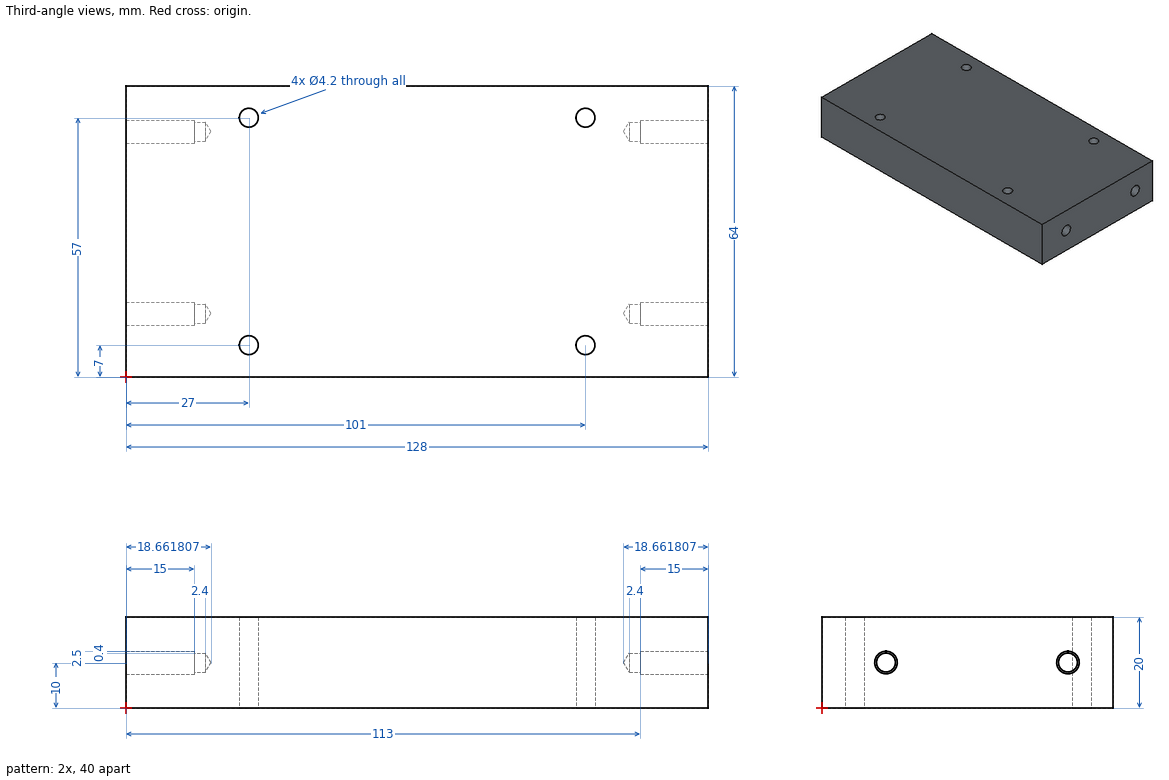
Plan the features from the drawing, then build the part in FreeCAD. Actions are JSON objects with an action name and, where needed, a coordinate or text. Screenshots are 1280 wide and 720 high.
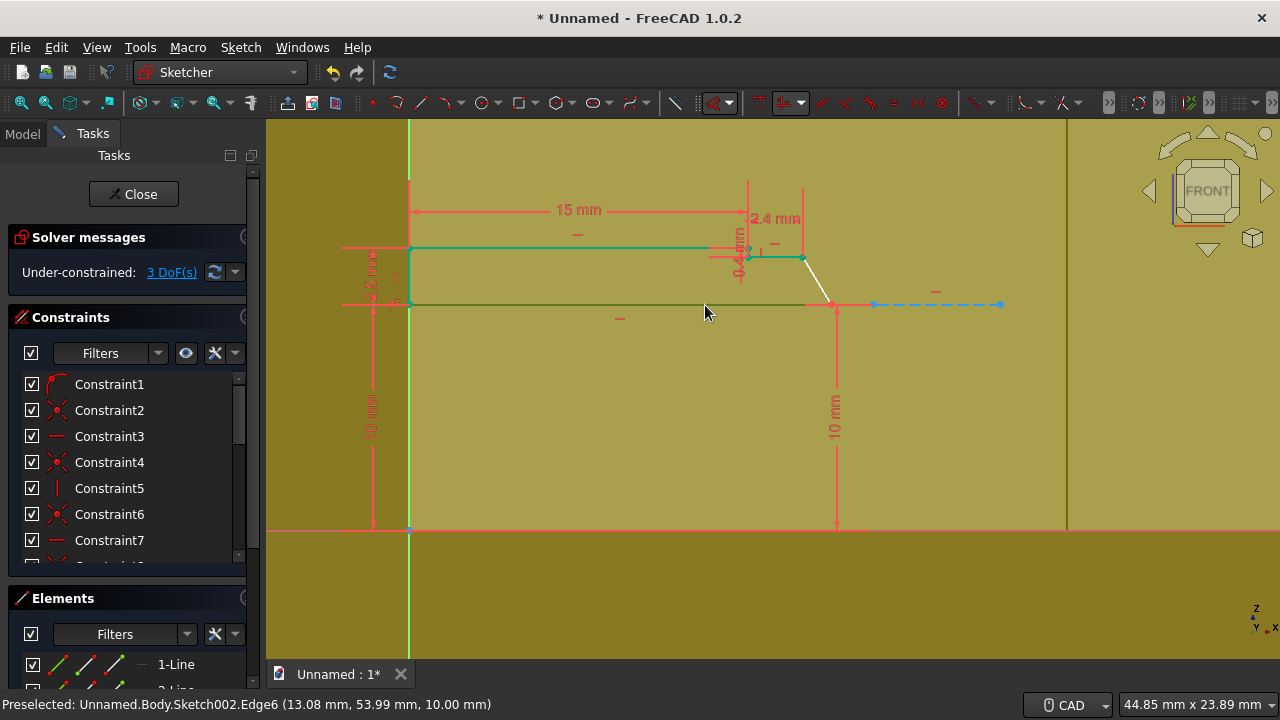
{"action": "left_click", "coordinate": [732, 104]}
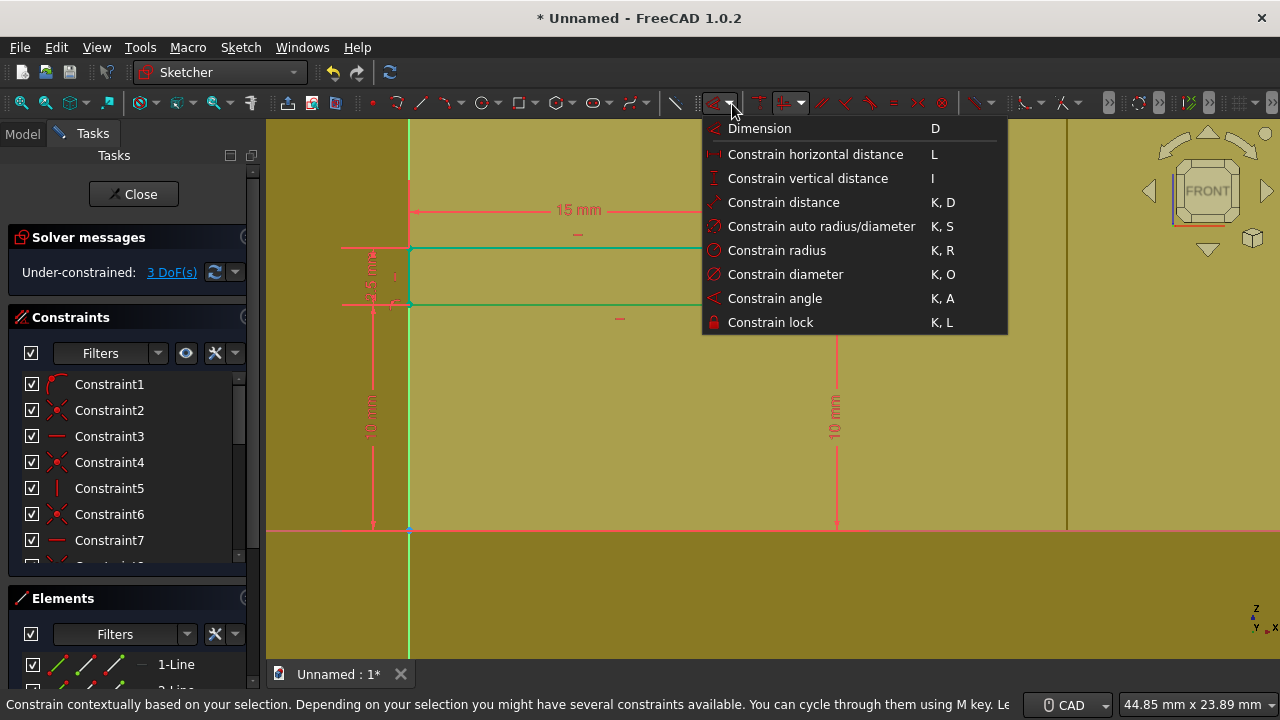
{"action": "left_click", "coordinate": [855, 154]}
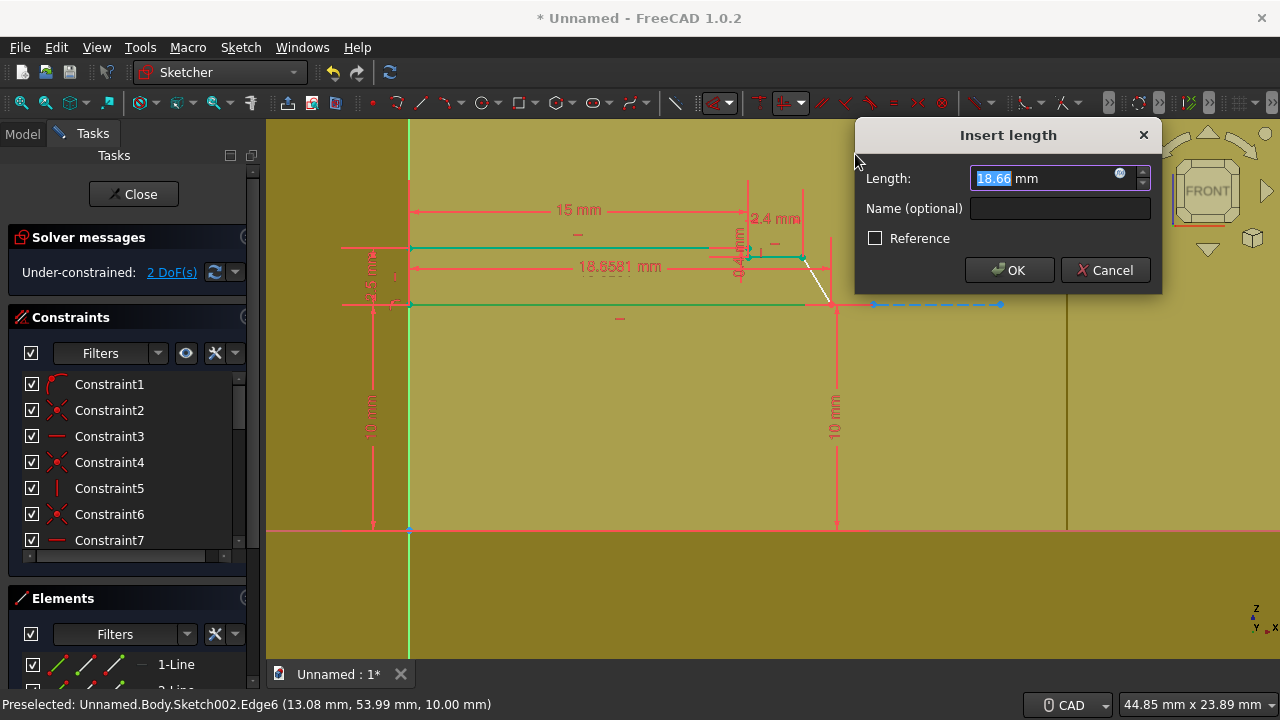
{"action": "type", "text": "18.661807"}
{"action": "key", "text": "Return"}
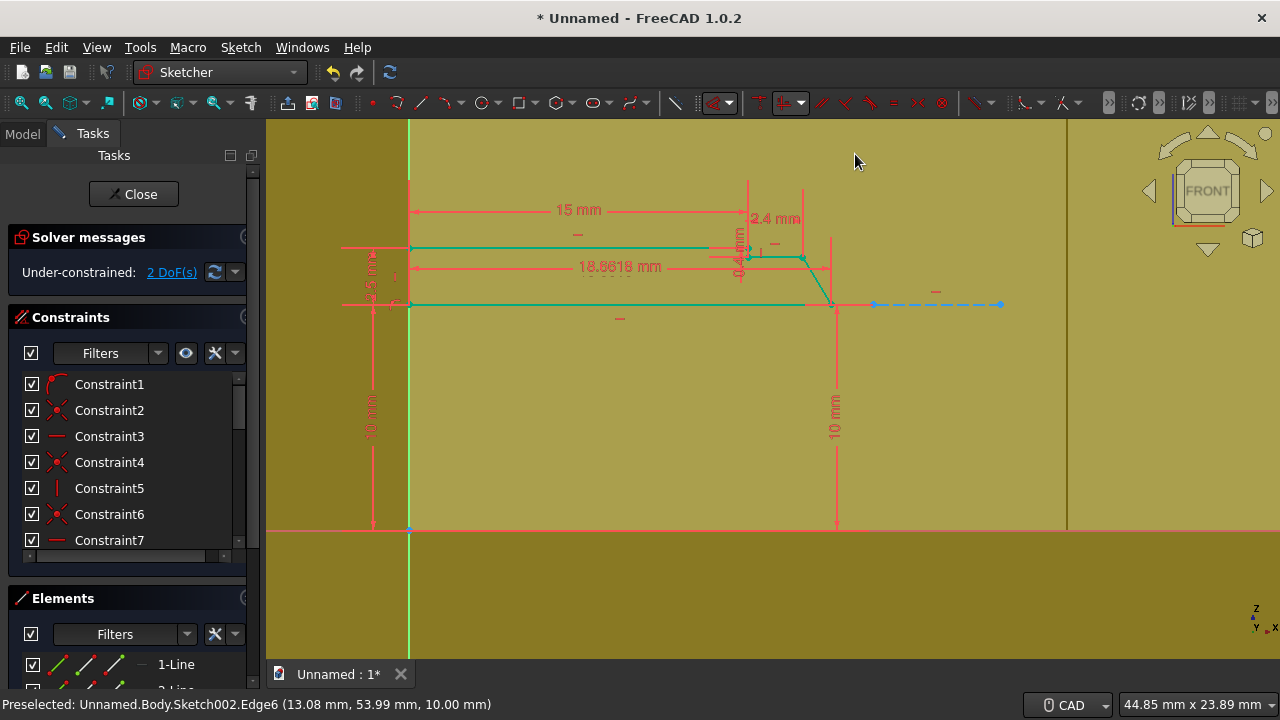
{"action": "left_click", "coordinate": [134, 194]}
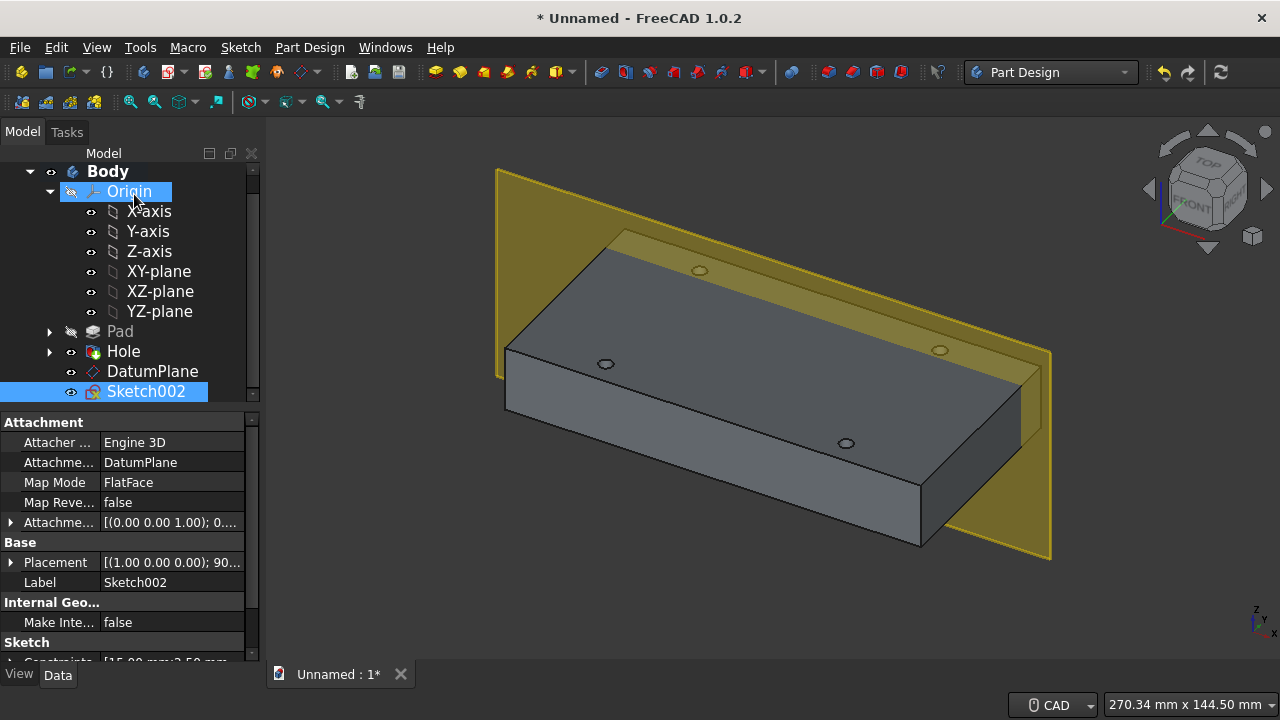
{"action": "left_click", "coordinate": [650, 72]}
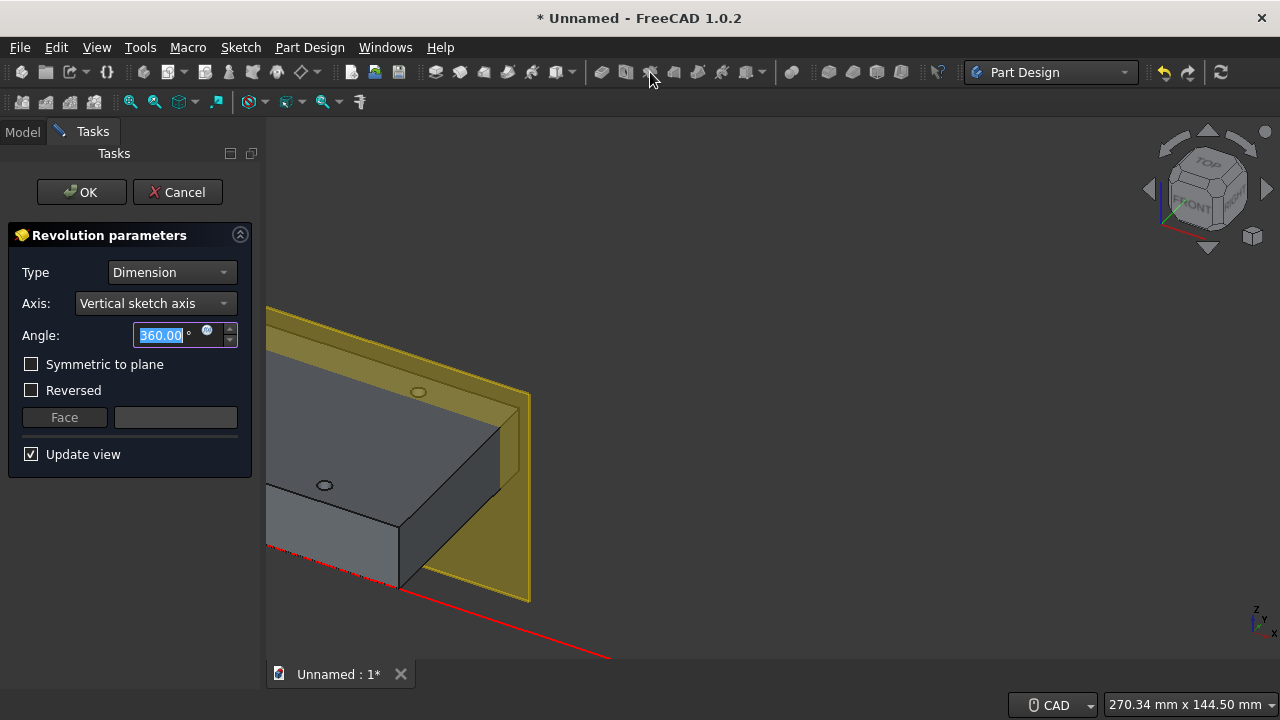
{"action": "left_click", "coordinate": [156, 304]}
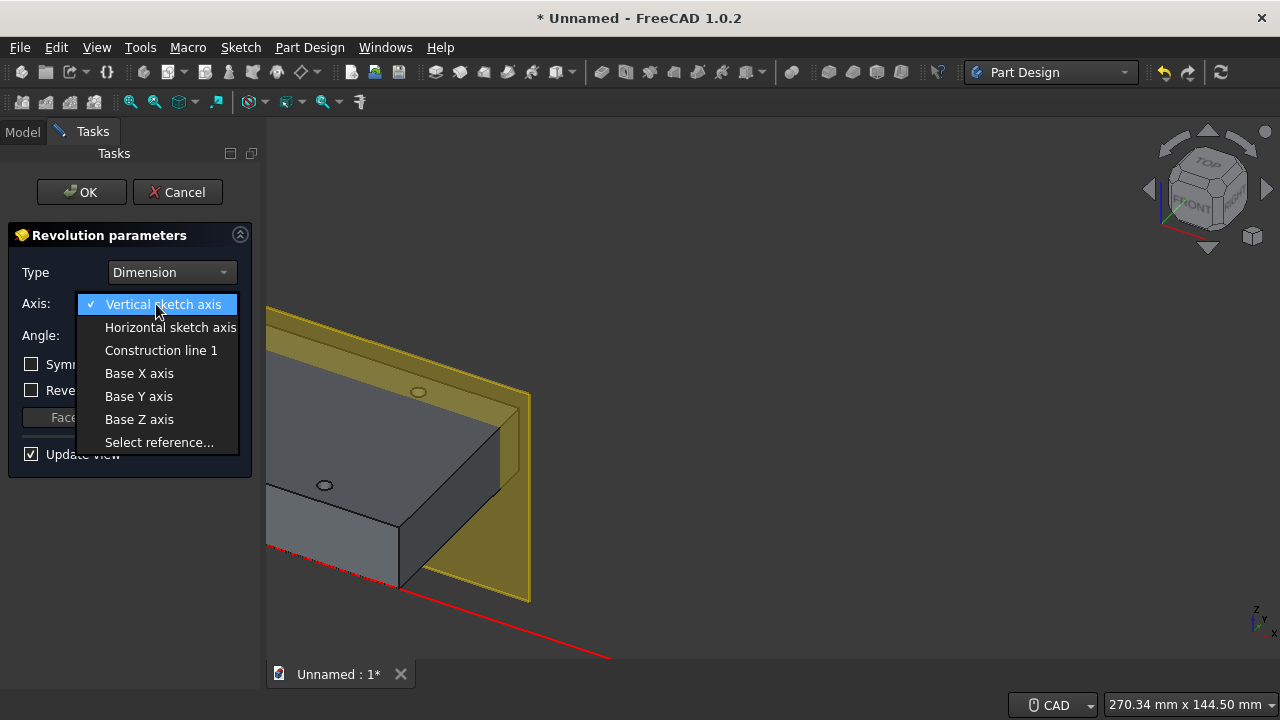
{"action": "left_click", "coordinate": [156, 350]}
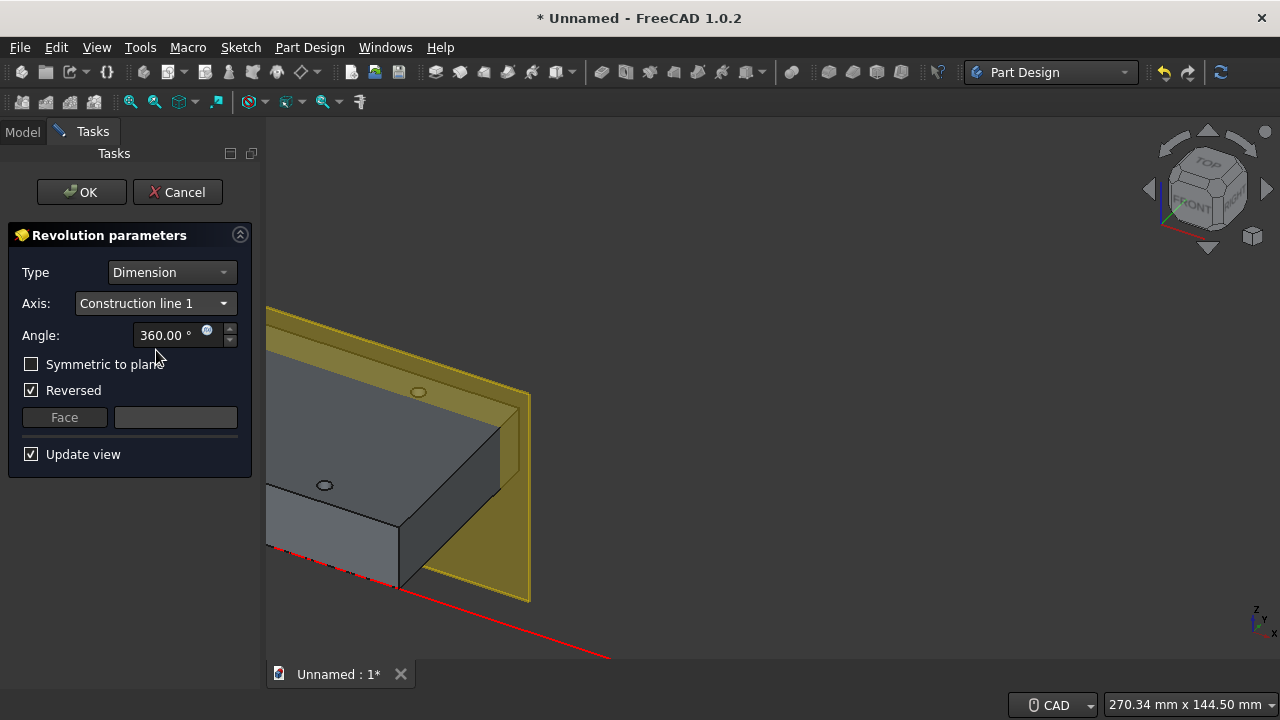
{"action": "left_click", "coordinate": [82, 192]}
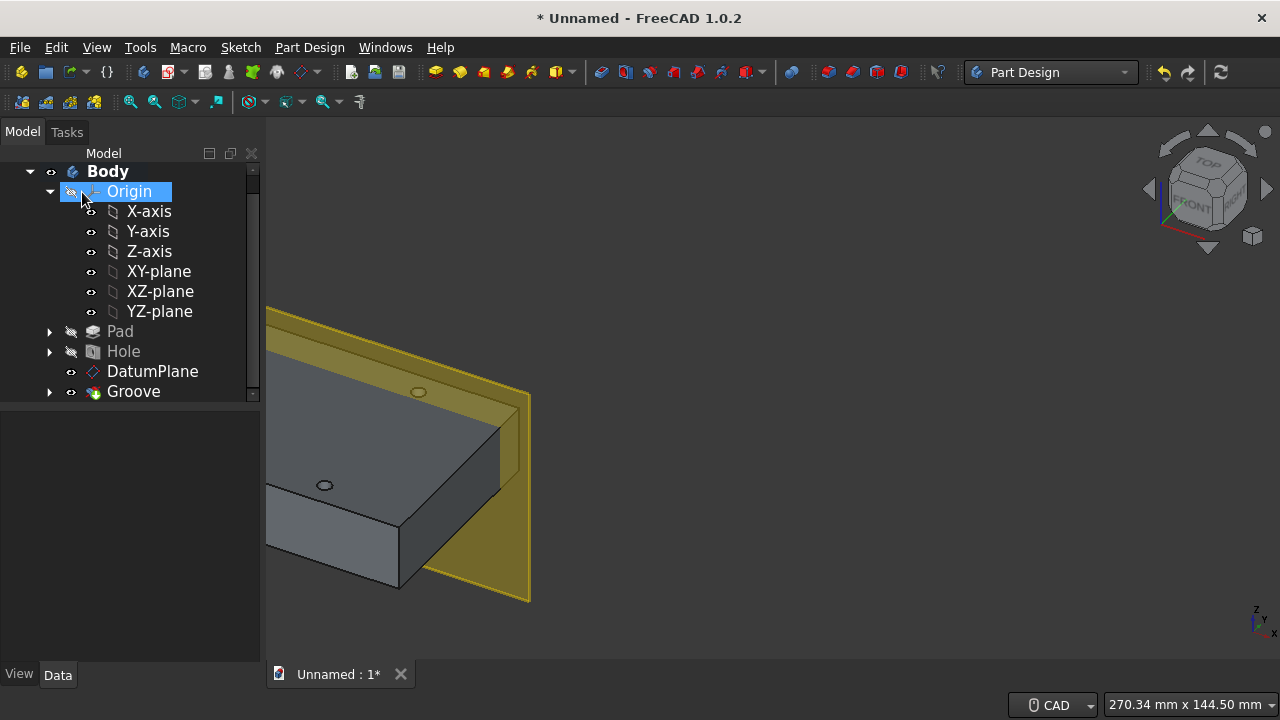
{"action": "left_click", "coordinate": [116, 372]}
{"action": "key", "text": "space"}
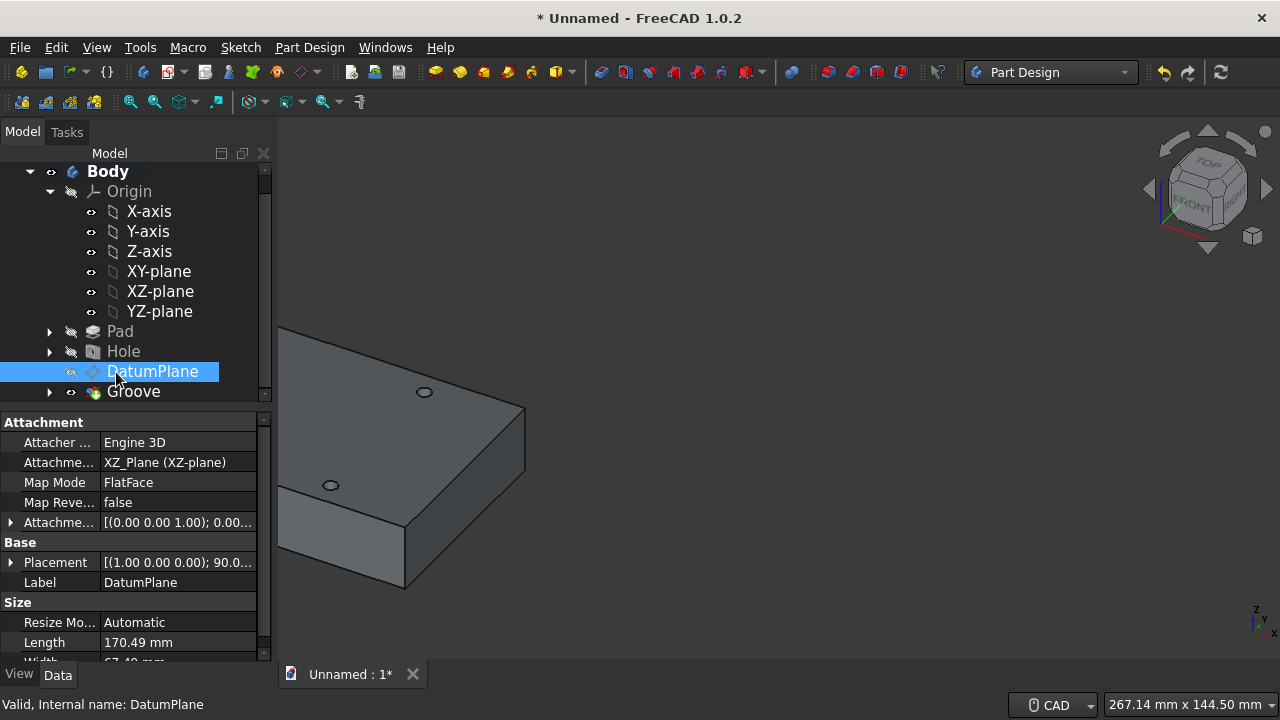
{"action": "left_click", "coordinate": [132, 102]}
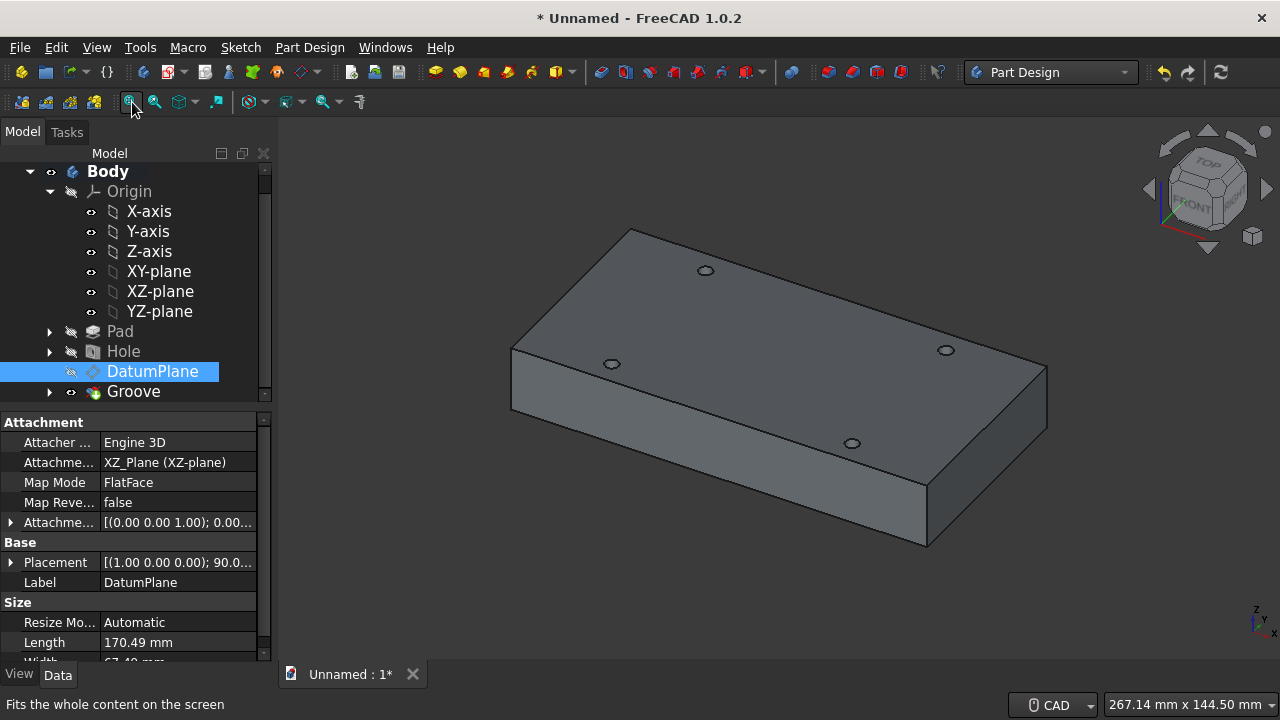
{"action": "left_click", "coordinate": [136, 312]}